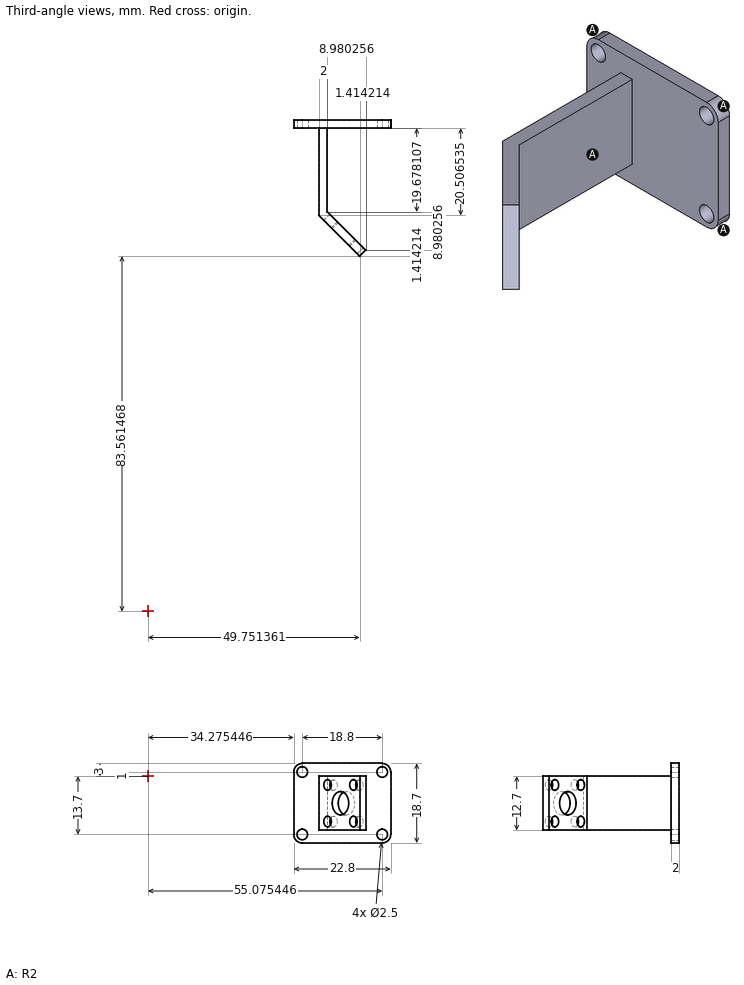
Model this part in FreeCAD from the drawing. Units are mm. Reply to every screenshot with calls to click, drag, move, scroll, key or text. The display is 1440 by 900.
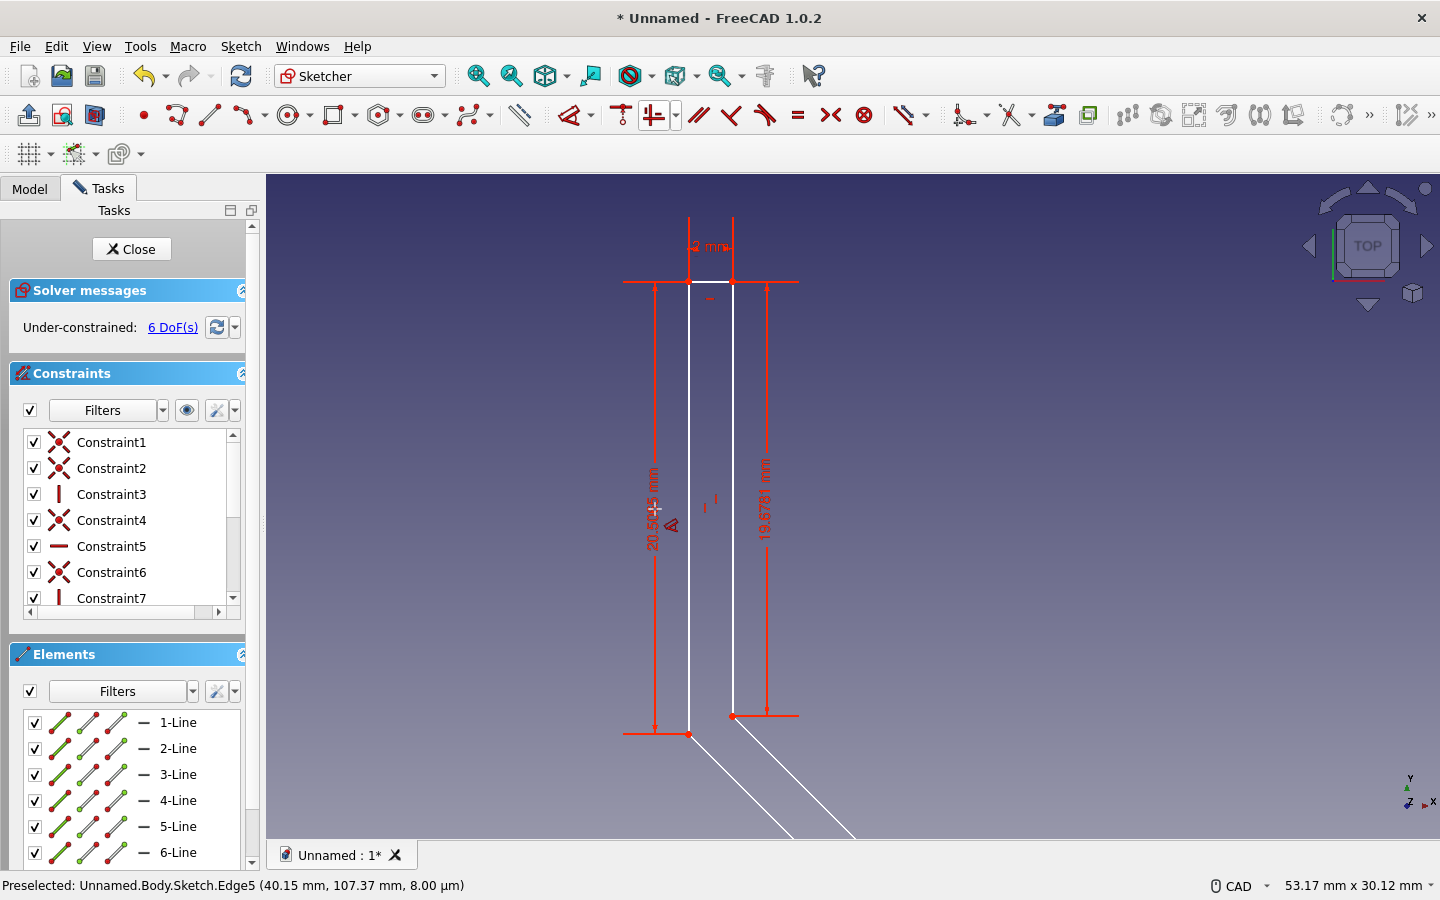
scroll(732, 290, down, 2)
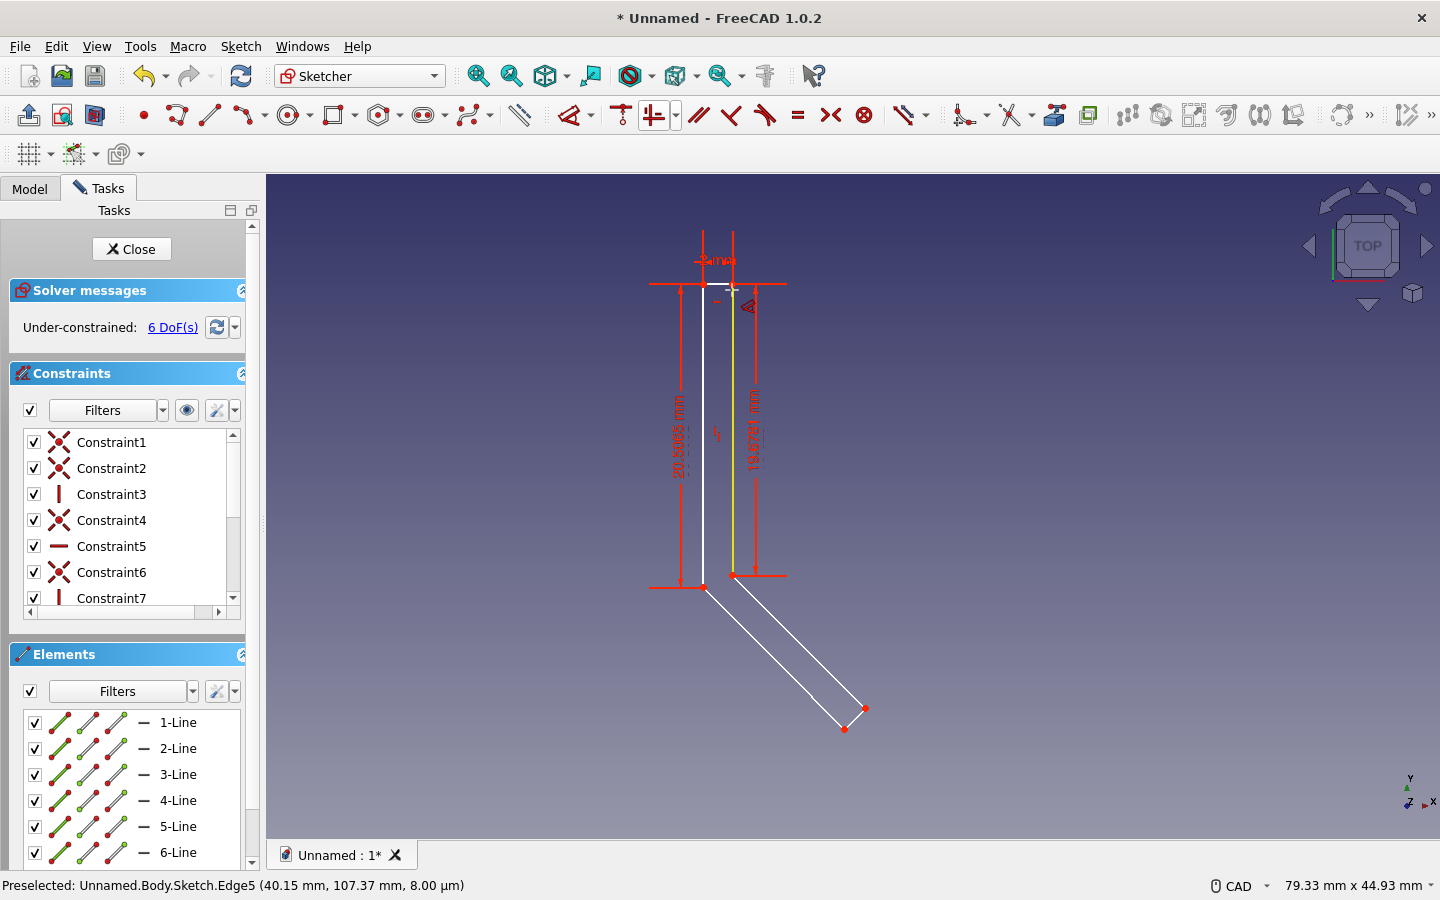
scroll(851, 723, up, 4)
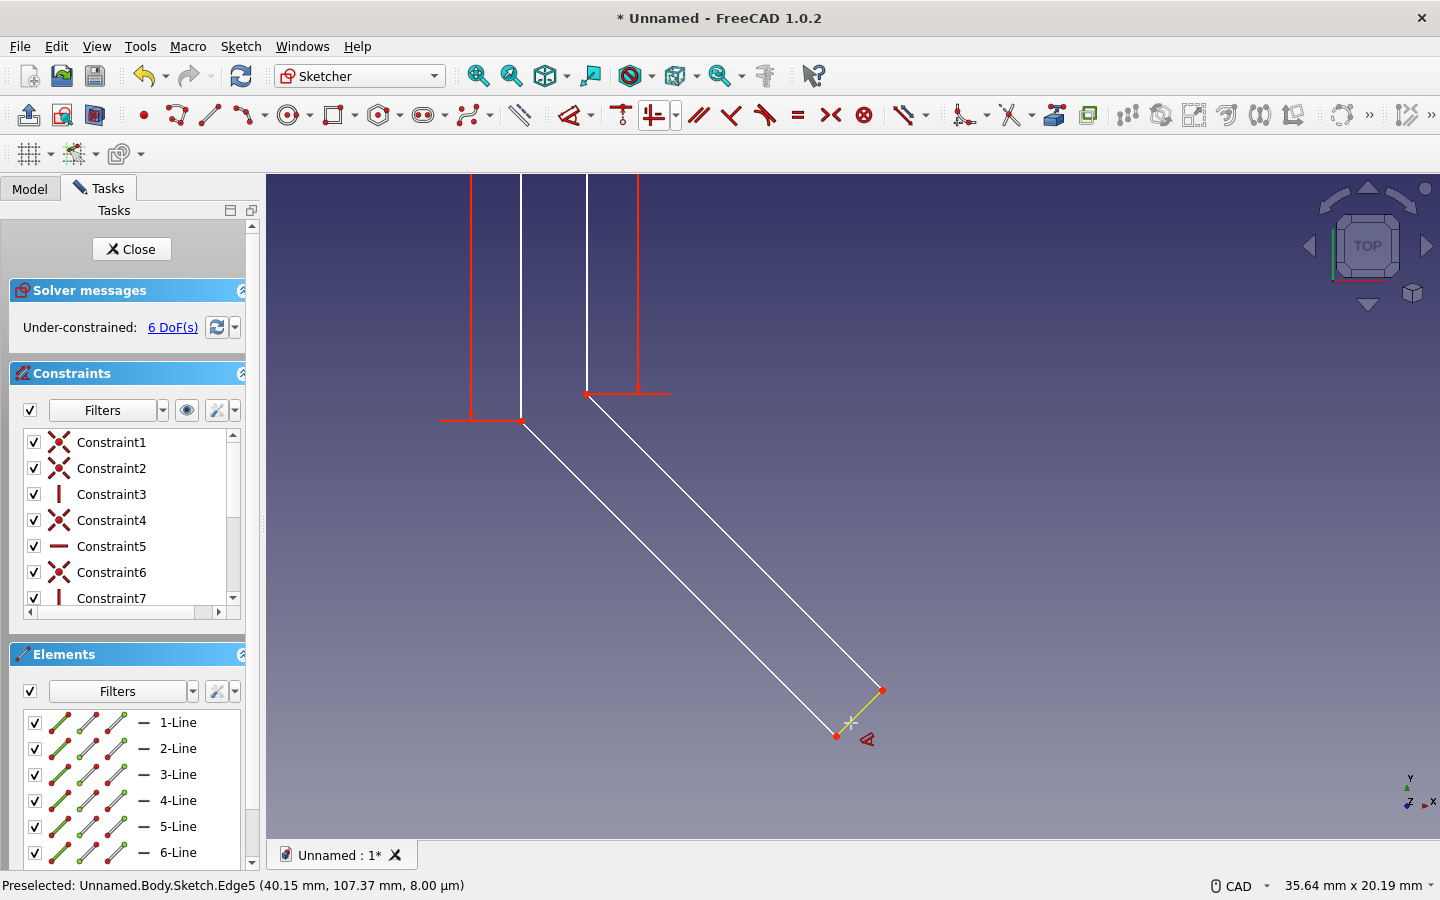
click(850, 723)
click(860, 771)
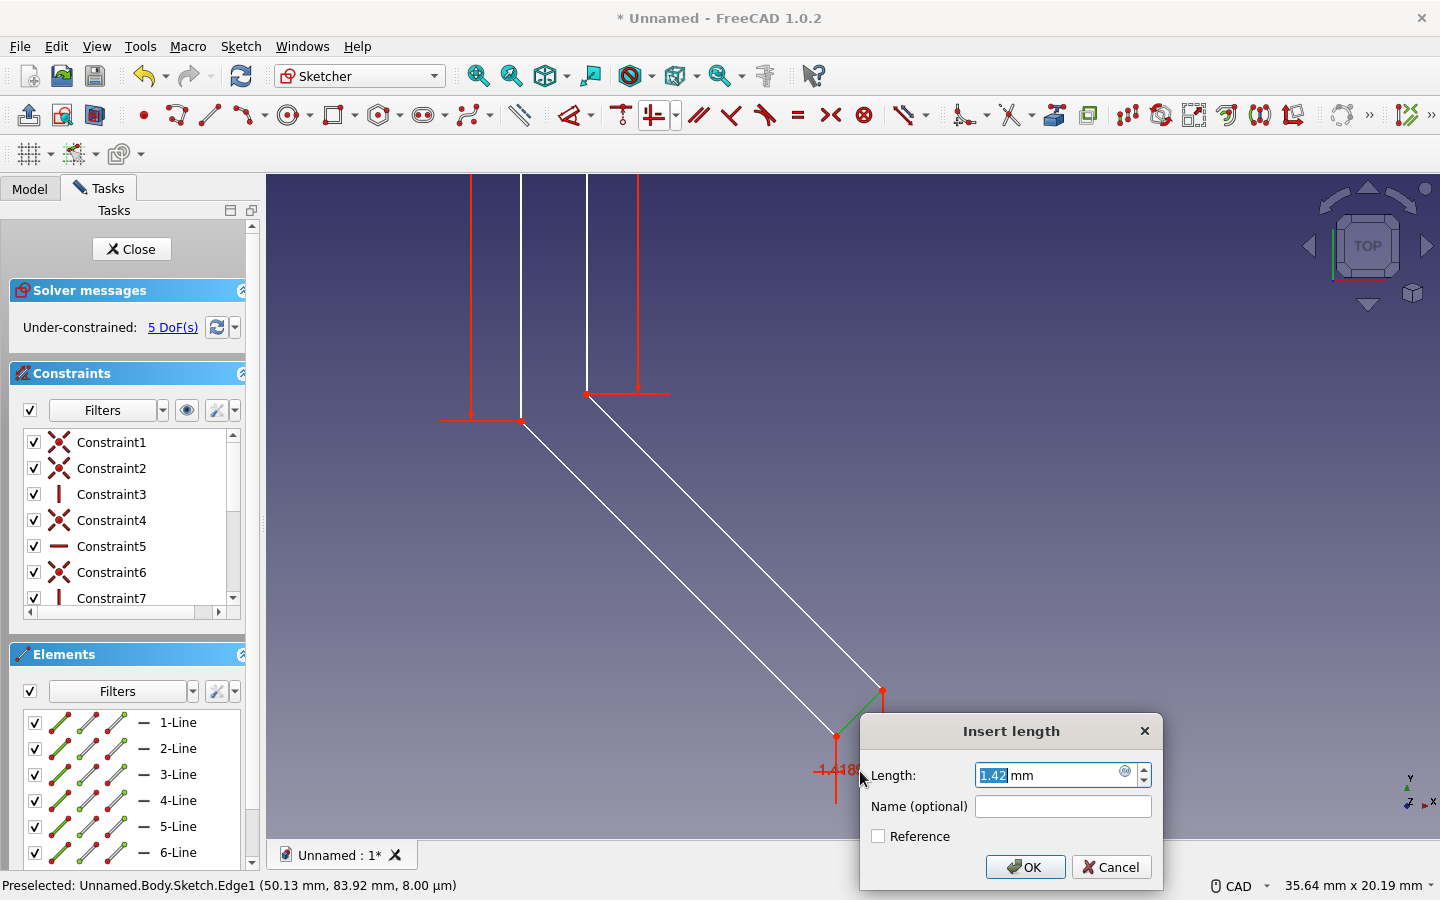
text(1.414214)
key(Return)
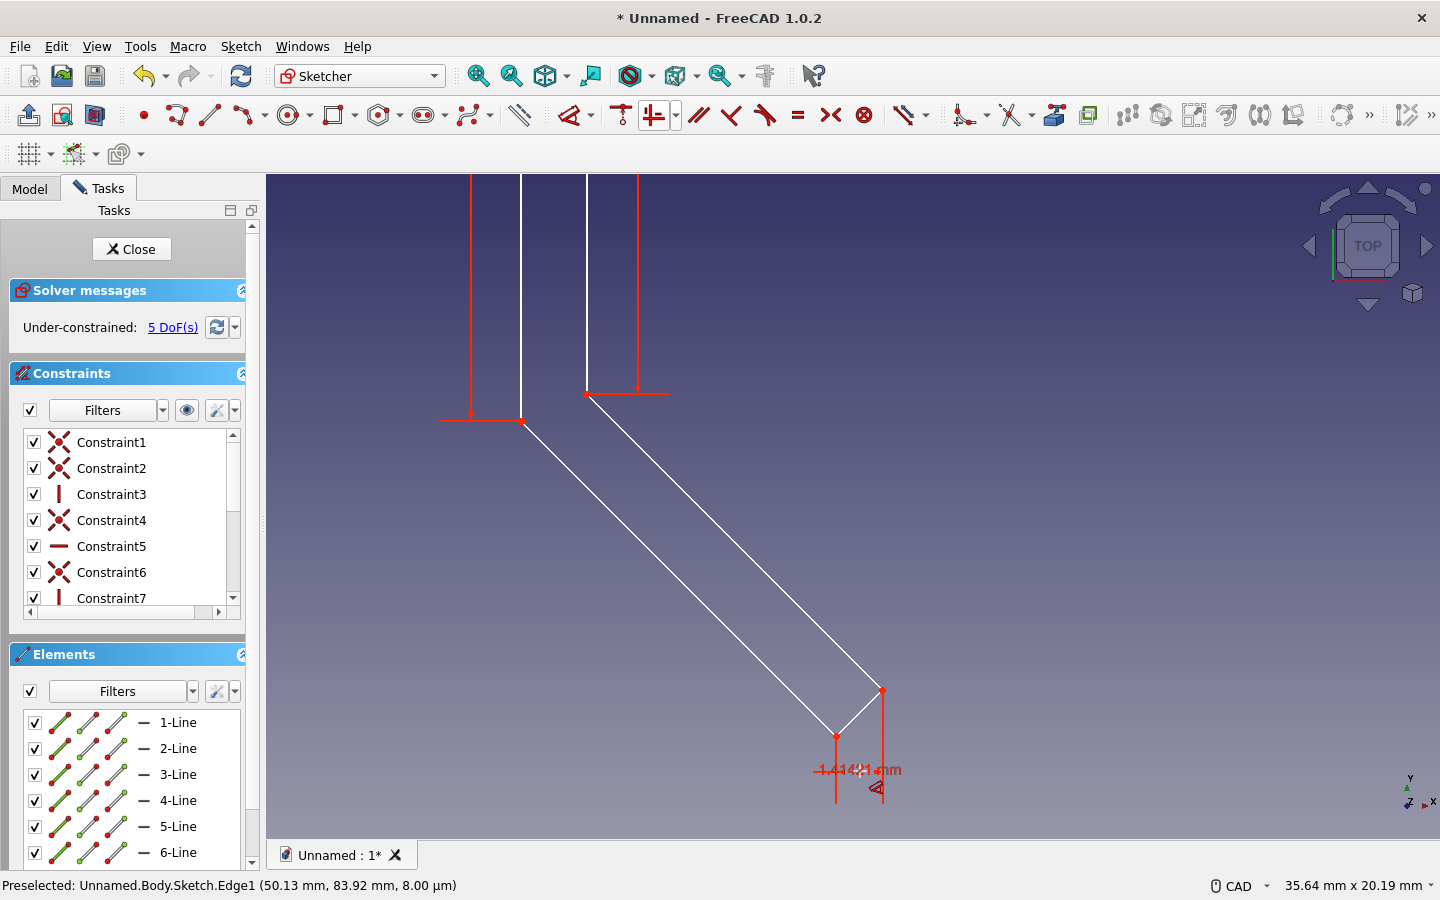
click(850, 723)
click(917, 713)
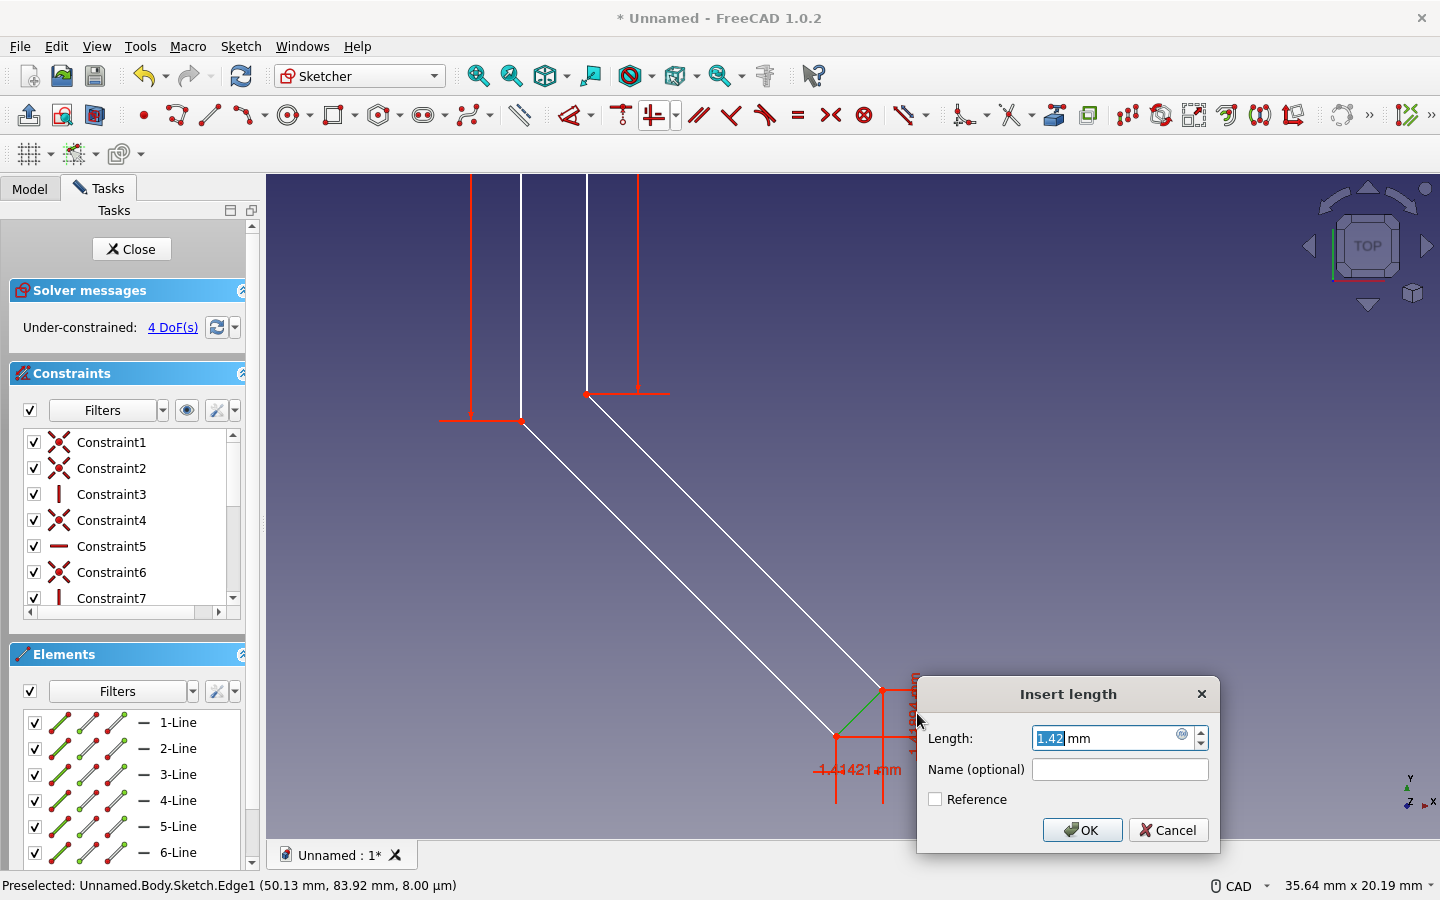
text(1.414214)
key(Return)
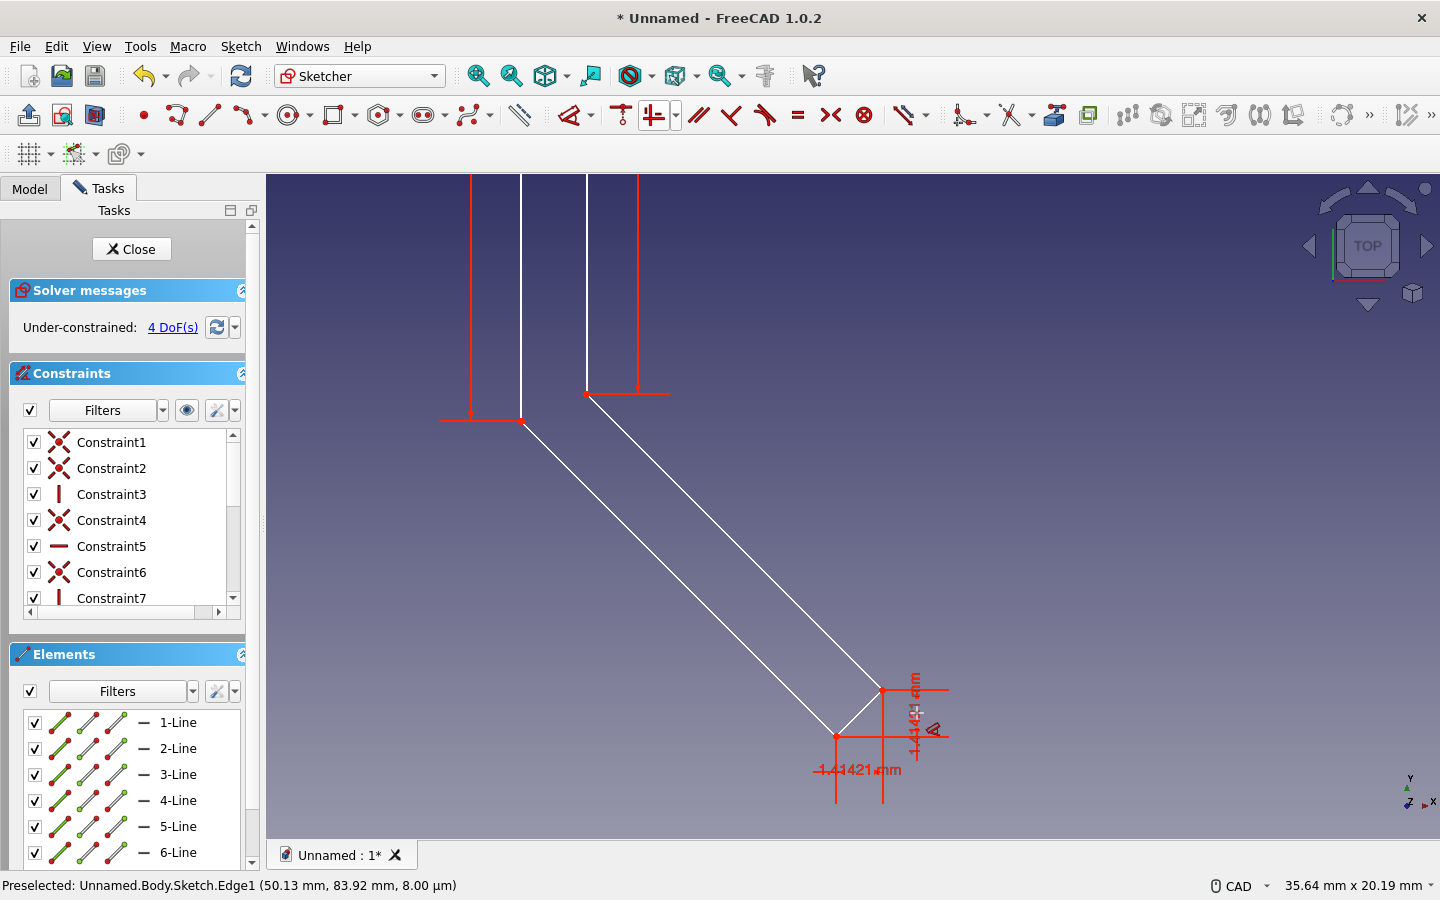
click(794, 601)
click(735, 724)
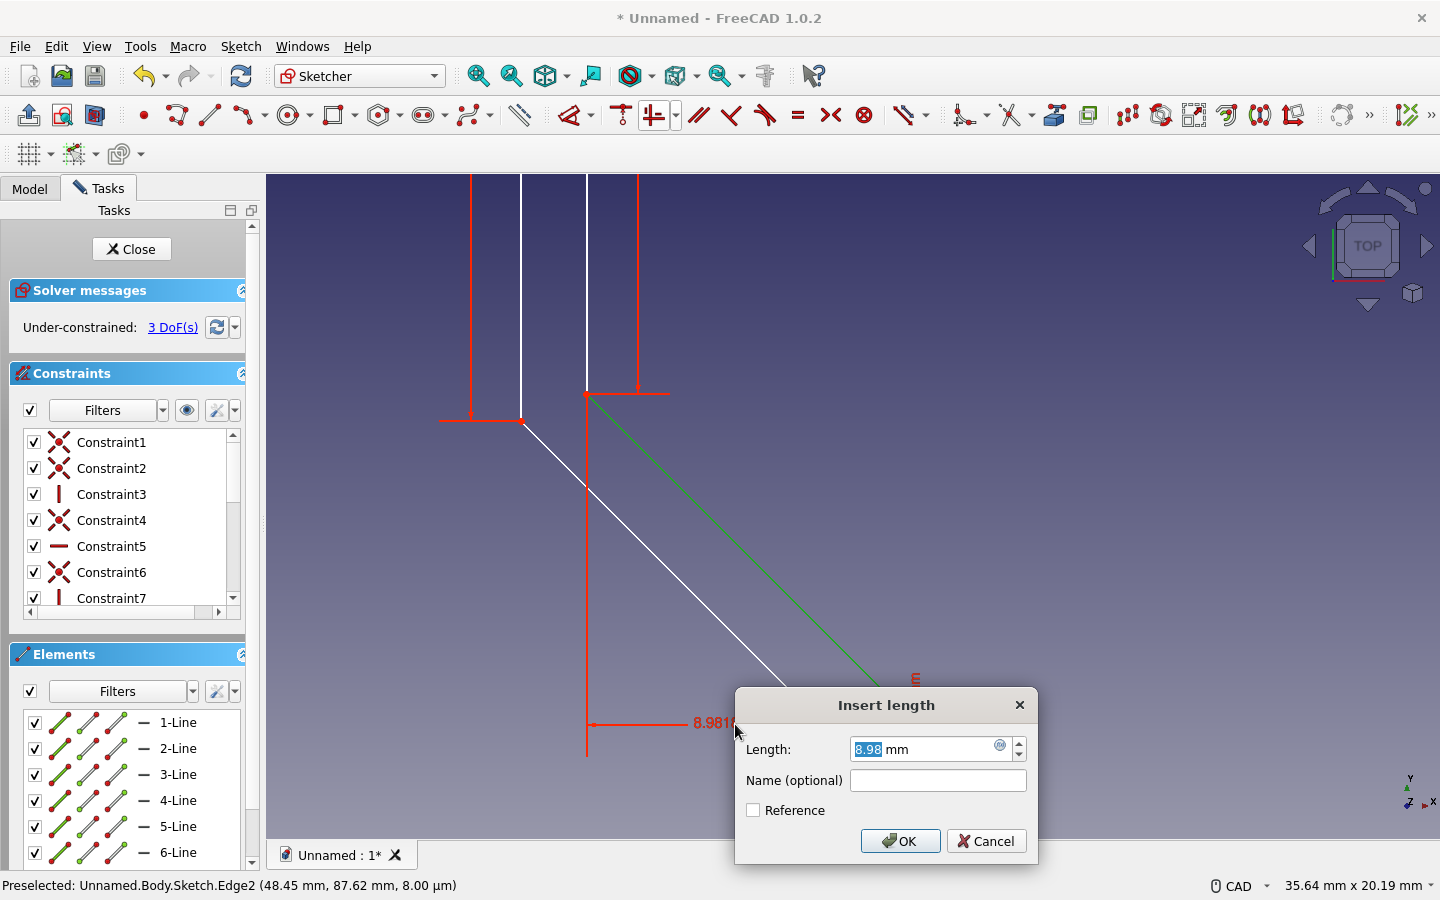
text(8.980256)
key(Return)